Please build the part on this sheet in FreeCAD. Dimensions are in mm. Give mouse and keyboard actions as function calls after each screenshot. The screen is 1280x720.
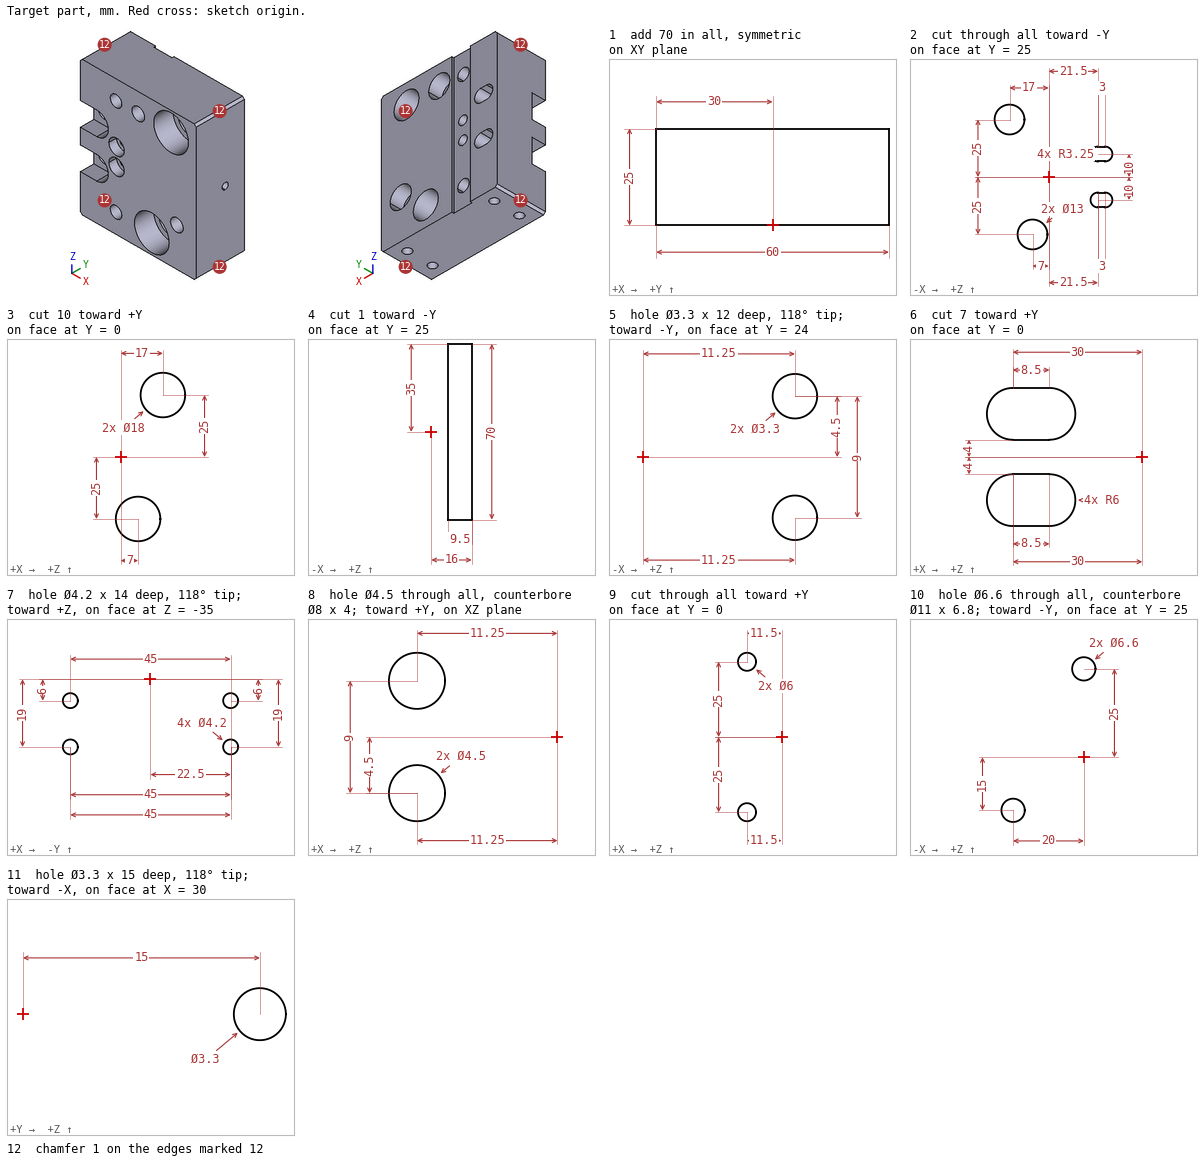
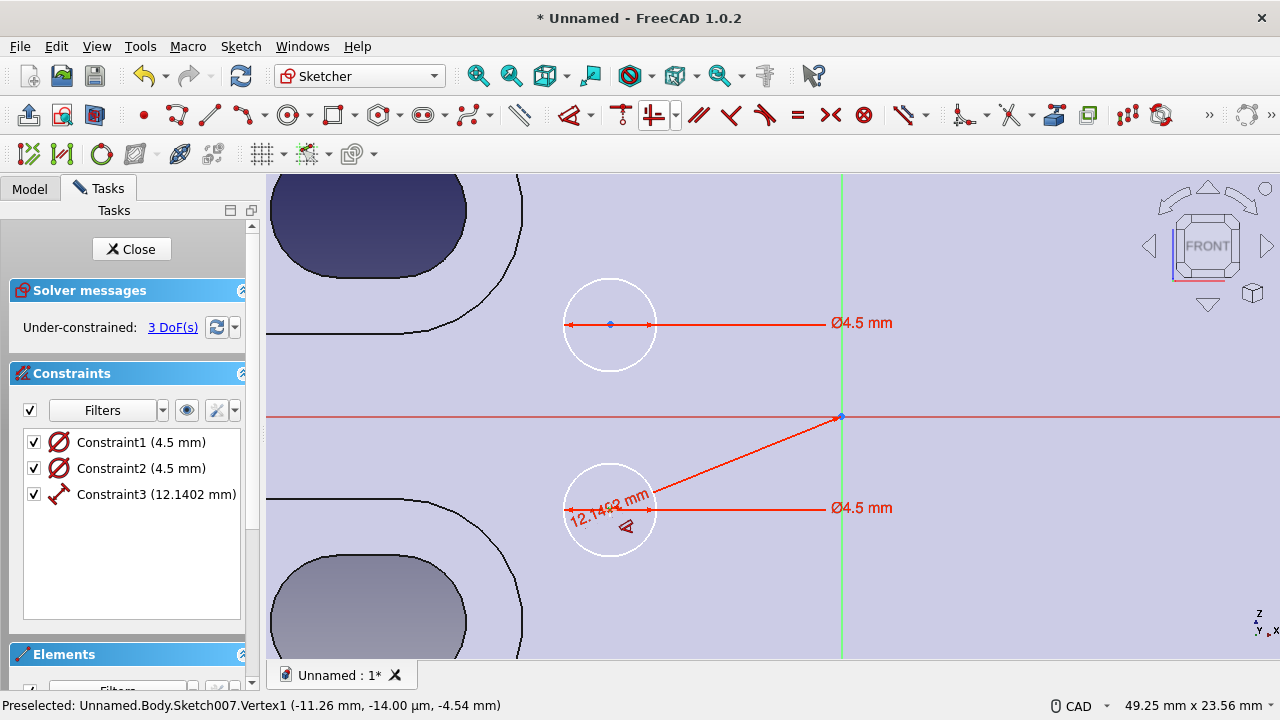
click(610, 325)
click(576, 375)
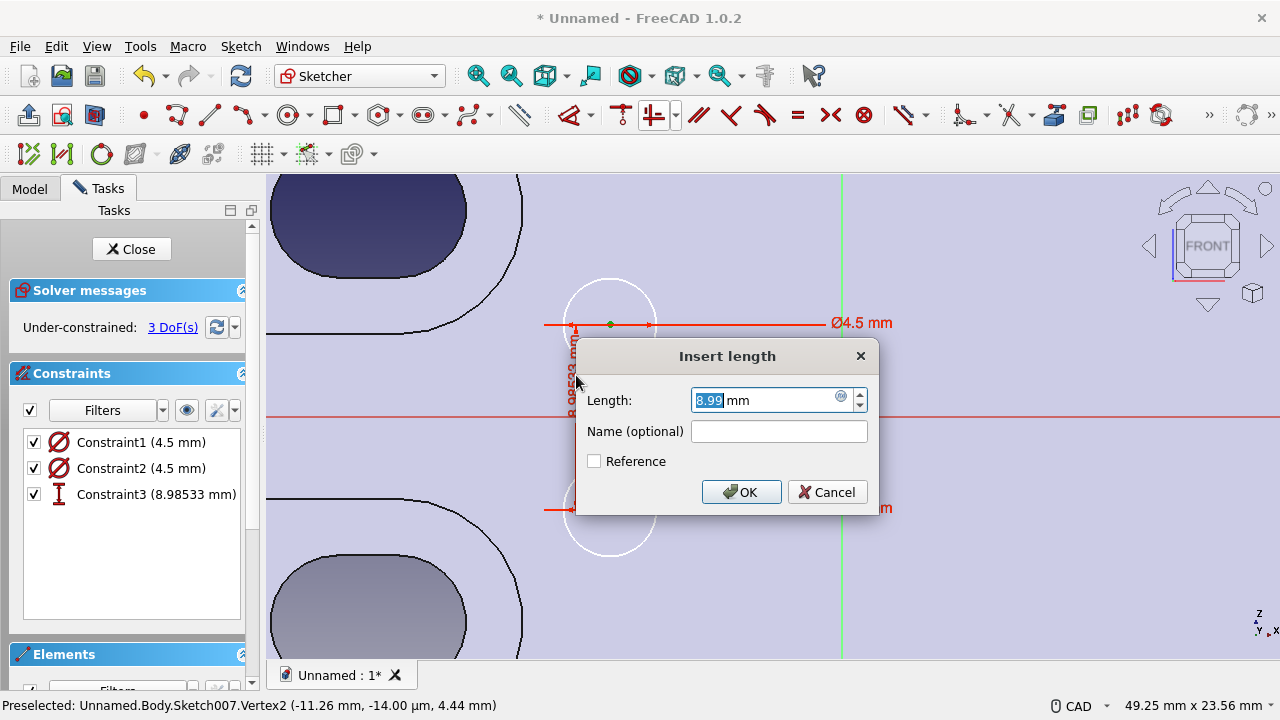
text(9)
key(Return)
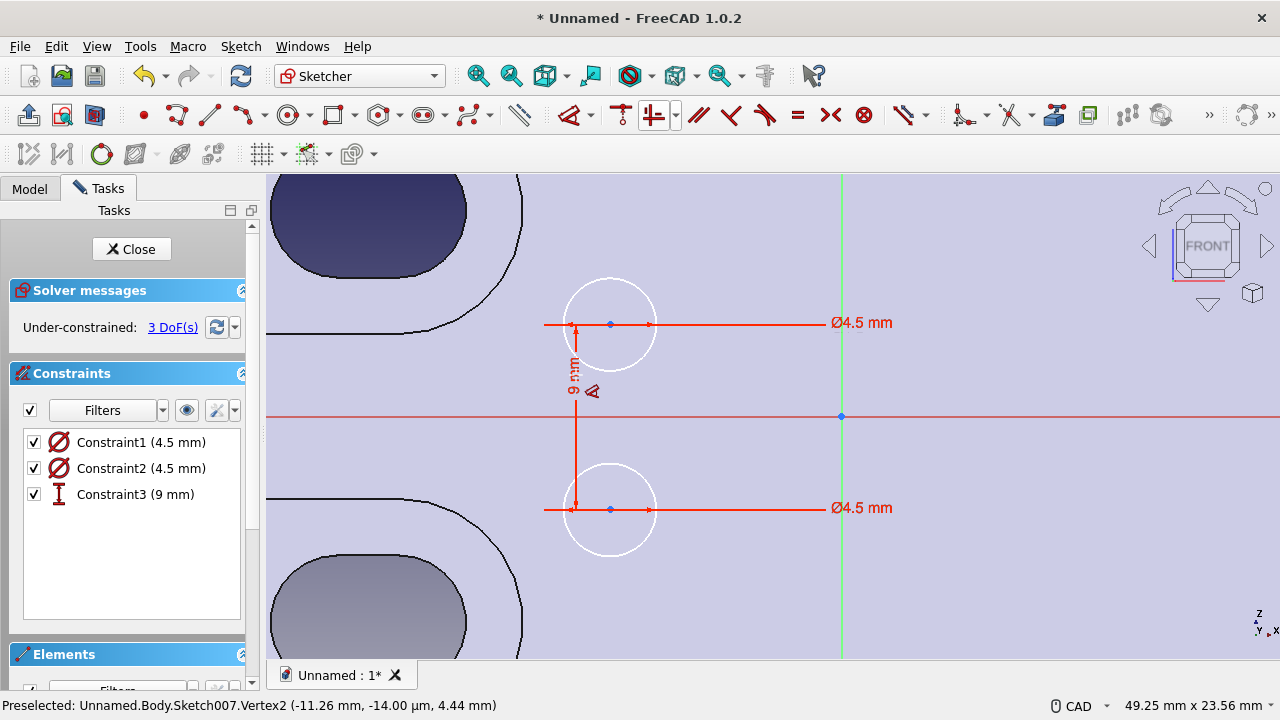
click(610, 510)
click(876, 463)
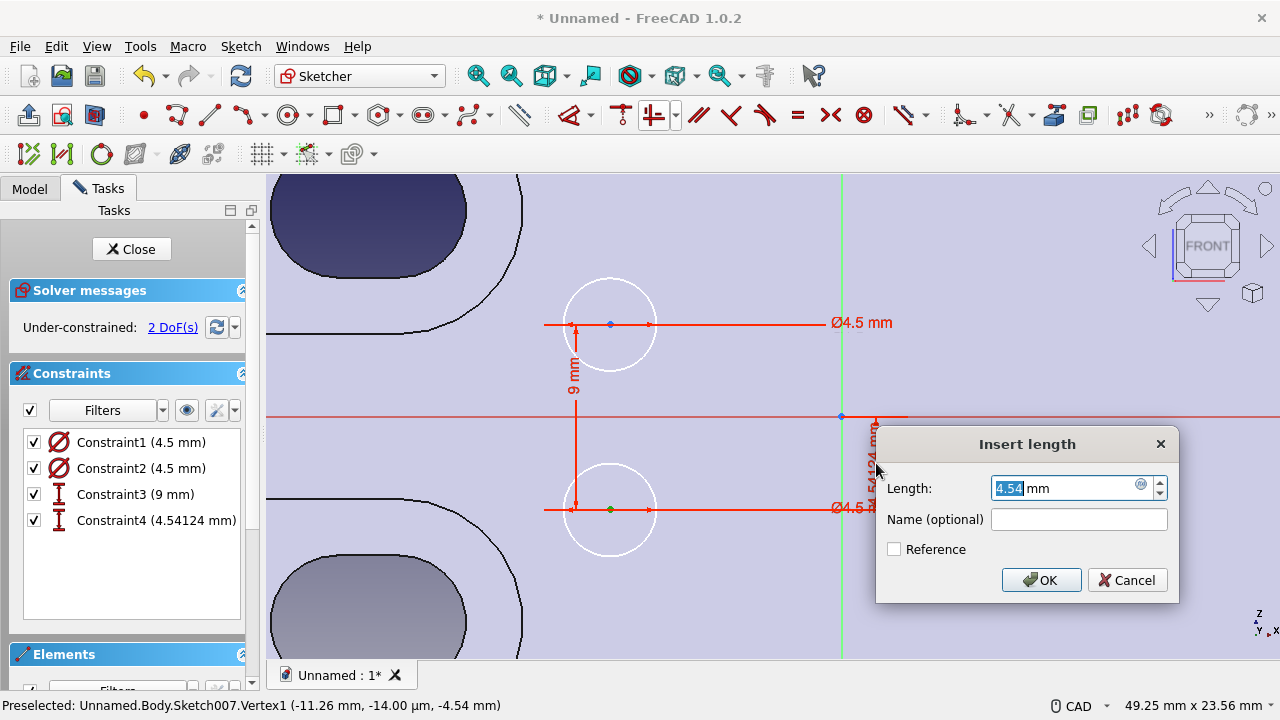
text(4.5)
key(Return)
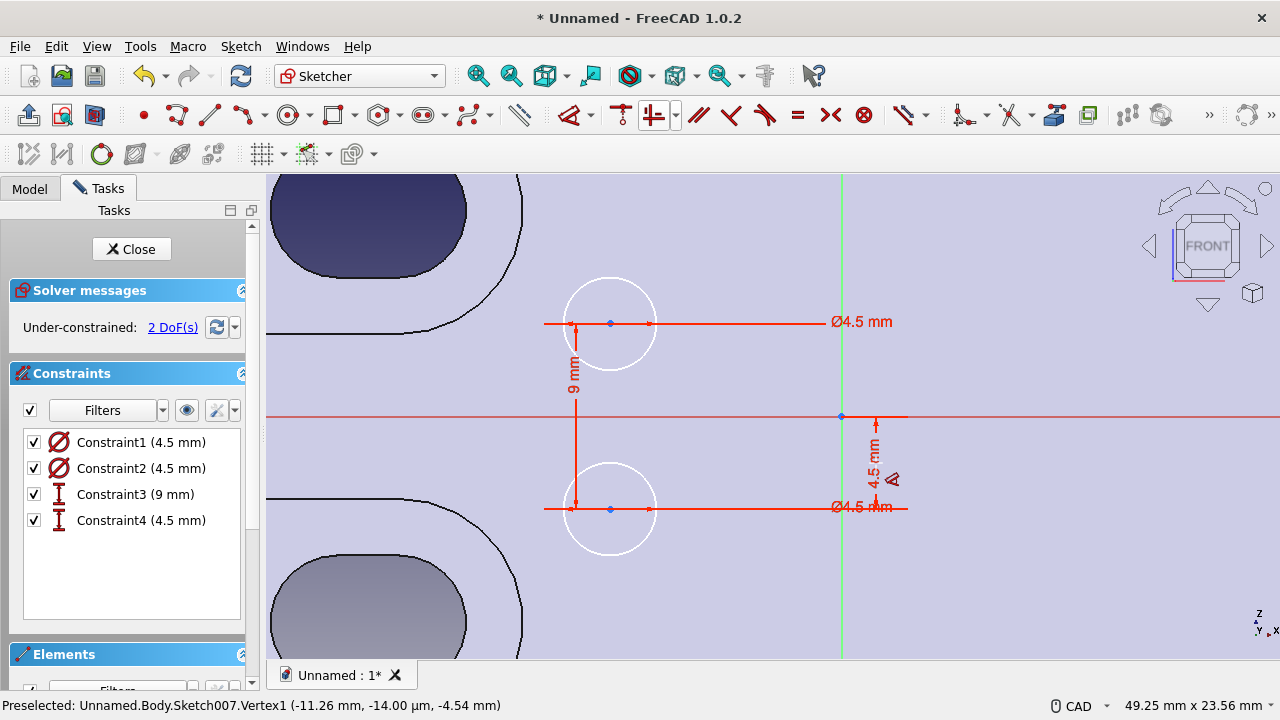
click(610, 509)
click(726, 543)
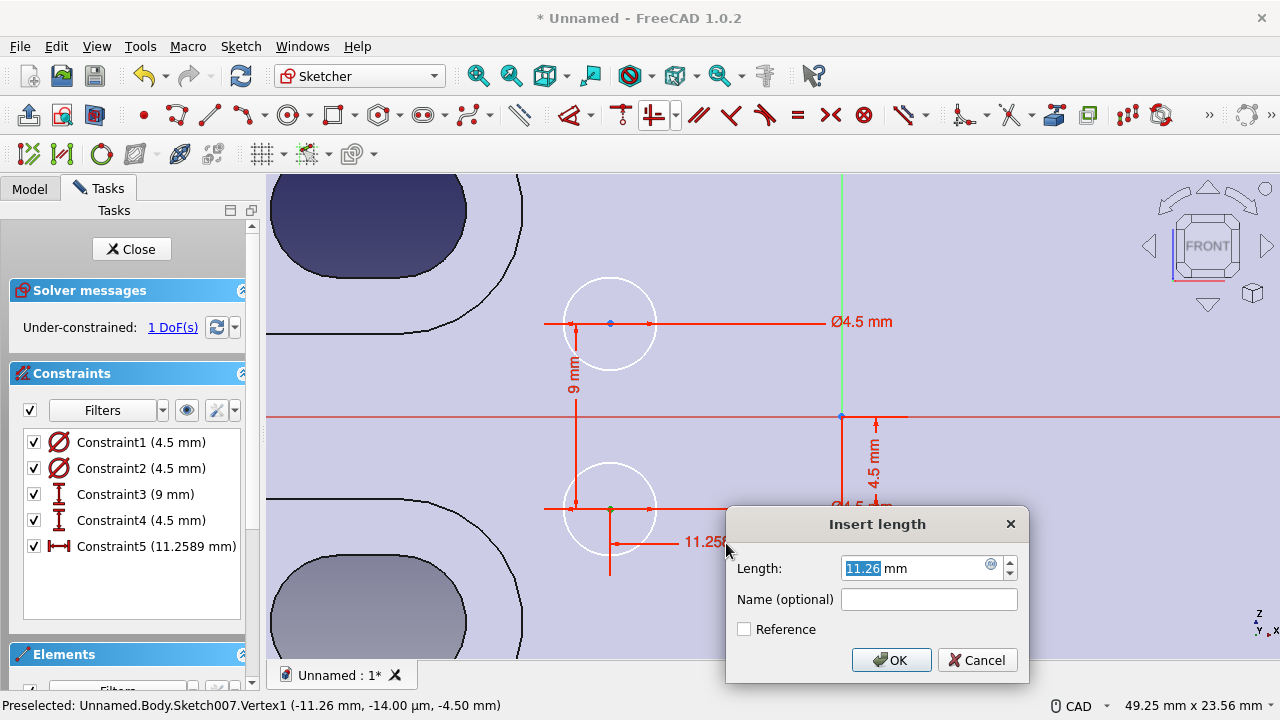
text(11.25)
key(Return)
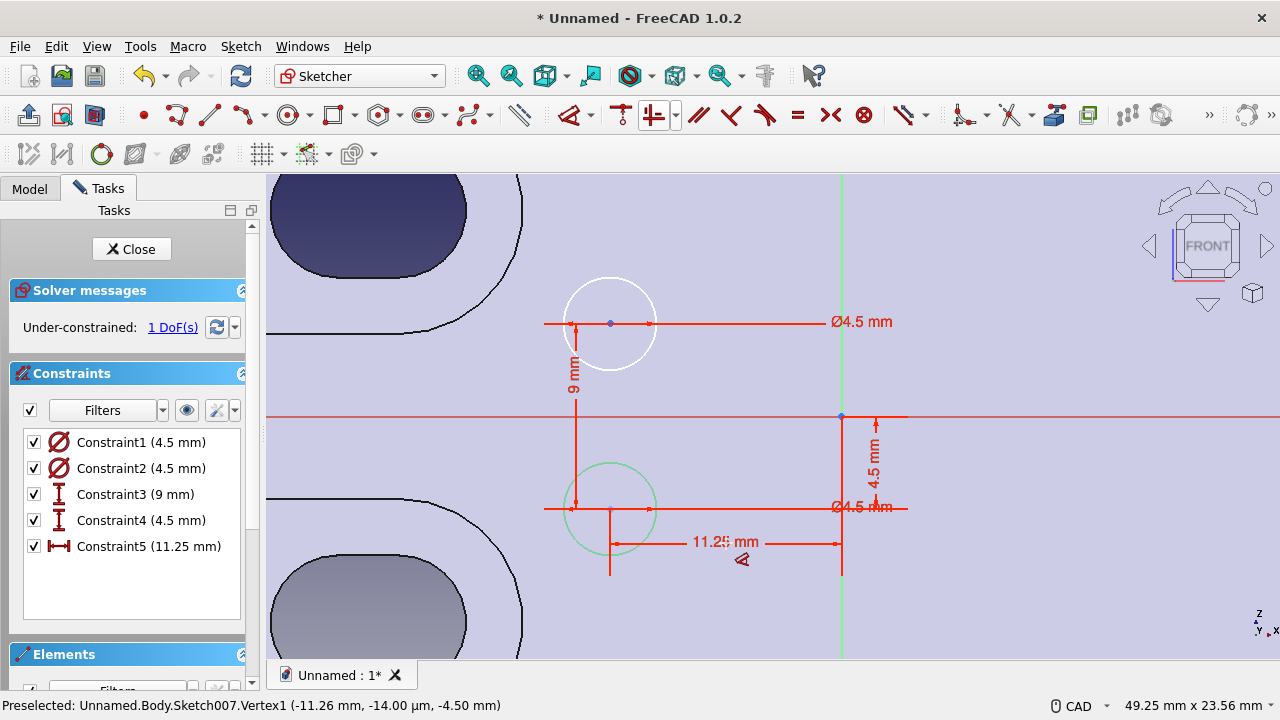
click(610, 324)
click(726, 290)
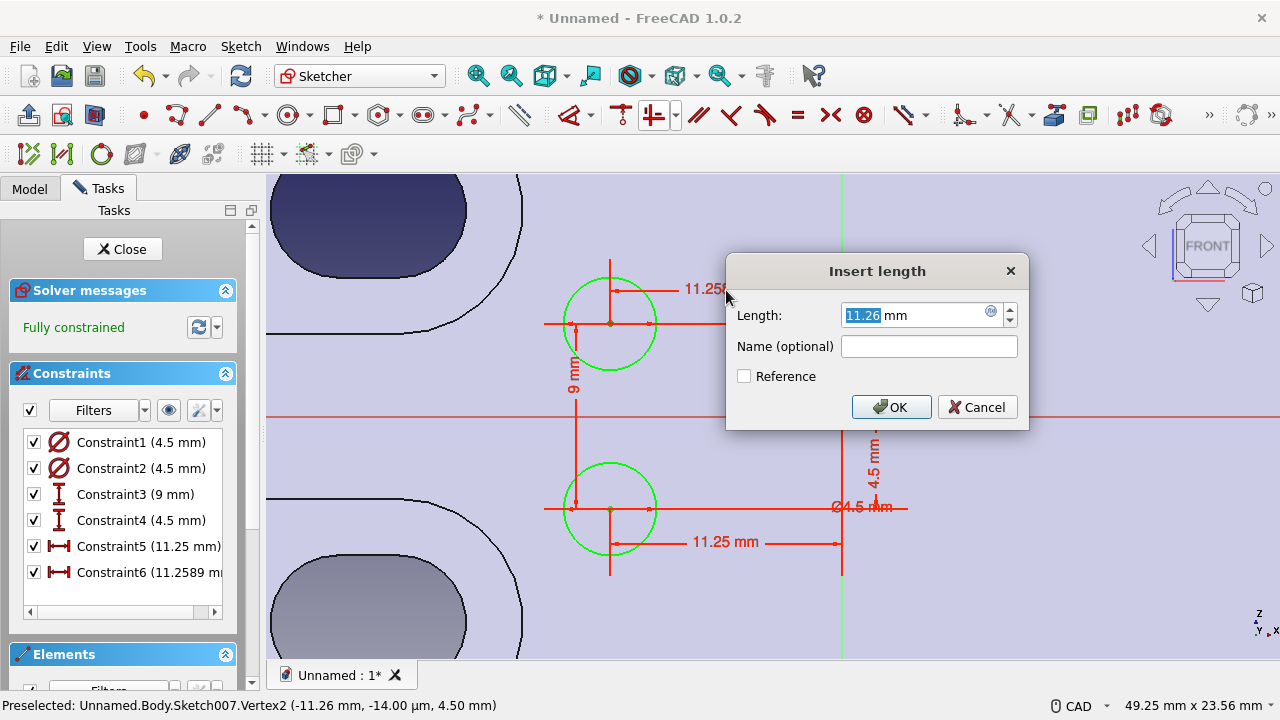
text(11.25)
key(Return)
key(Escape)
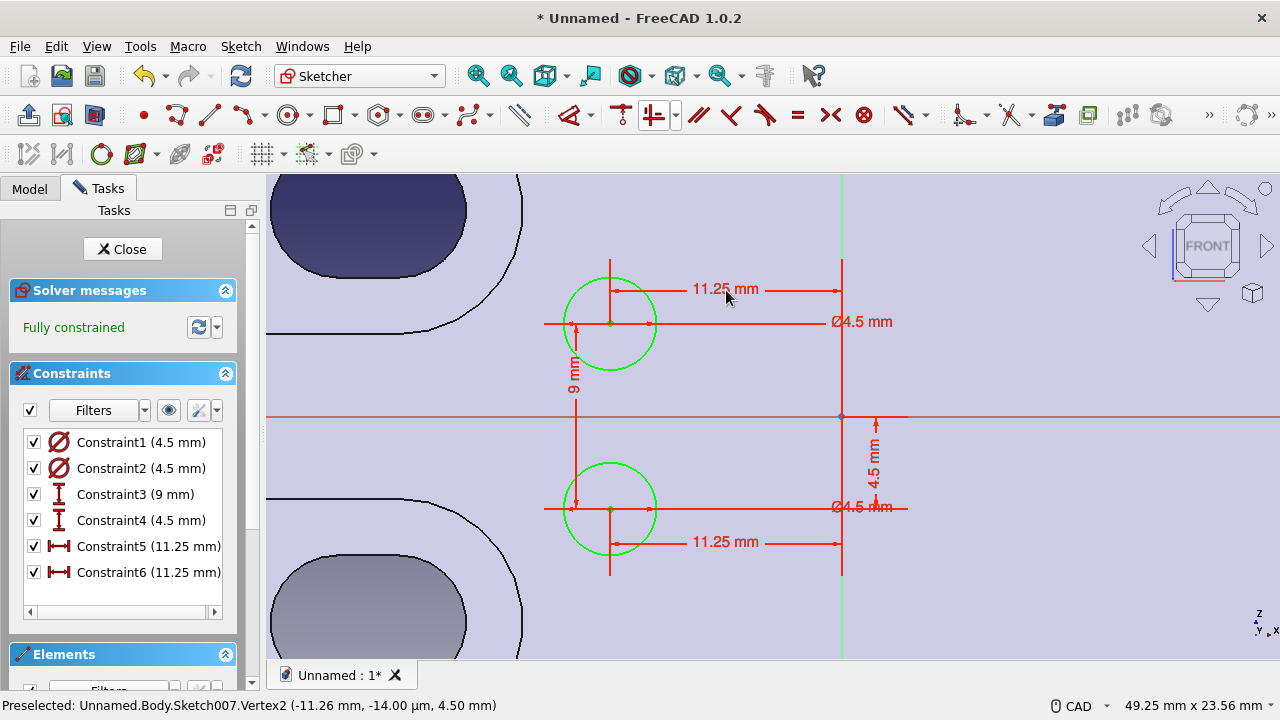
click(123, 249)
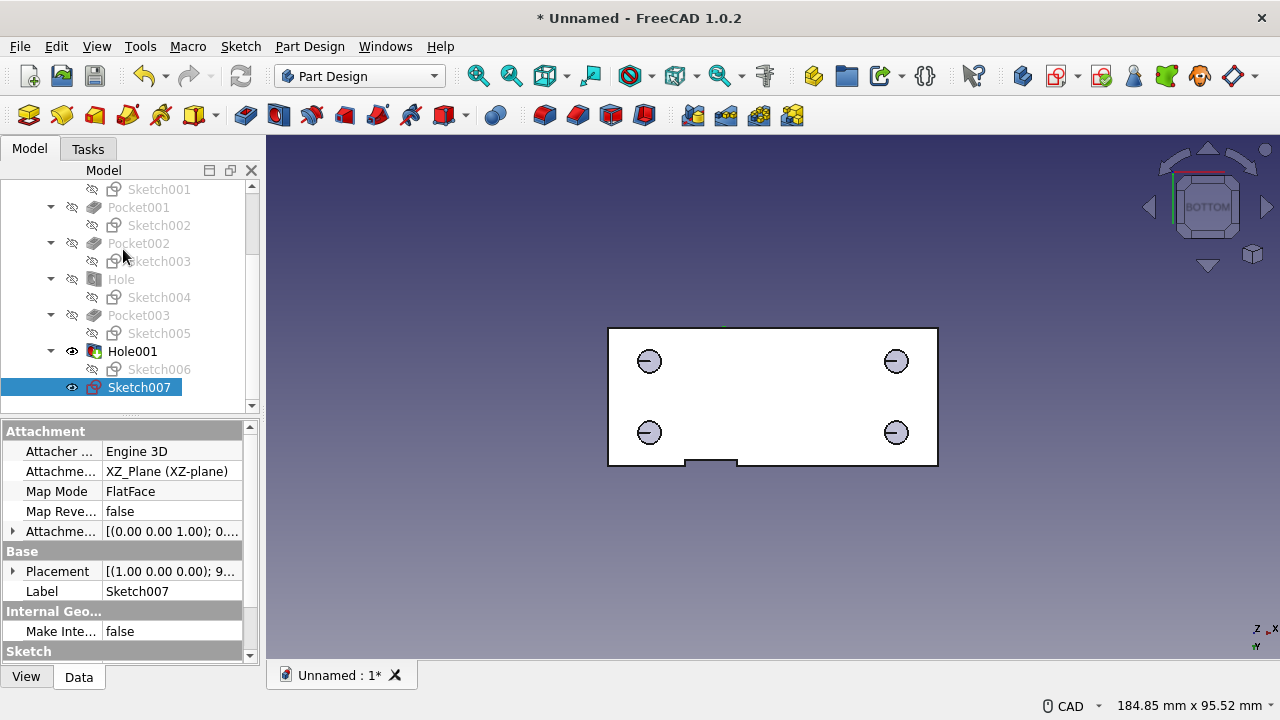
click(279, 116)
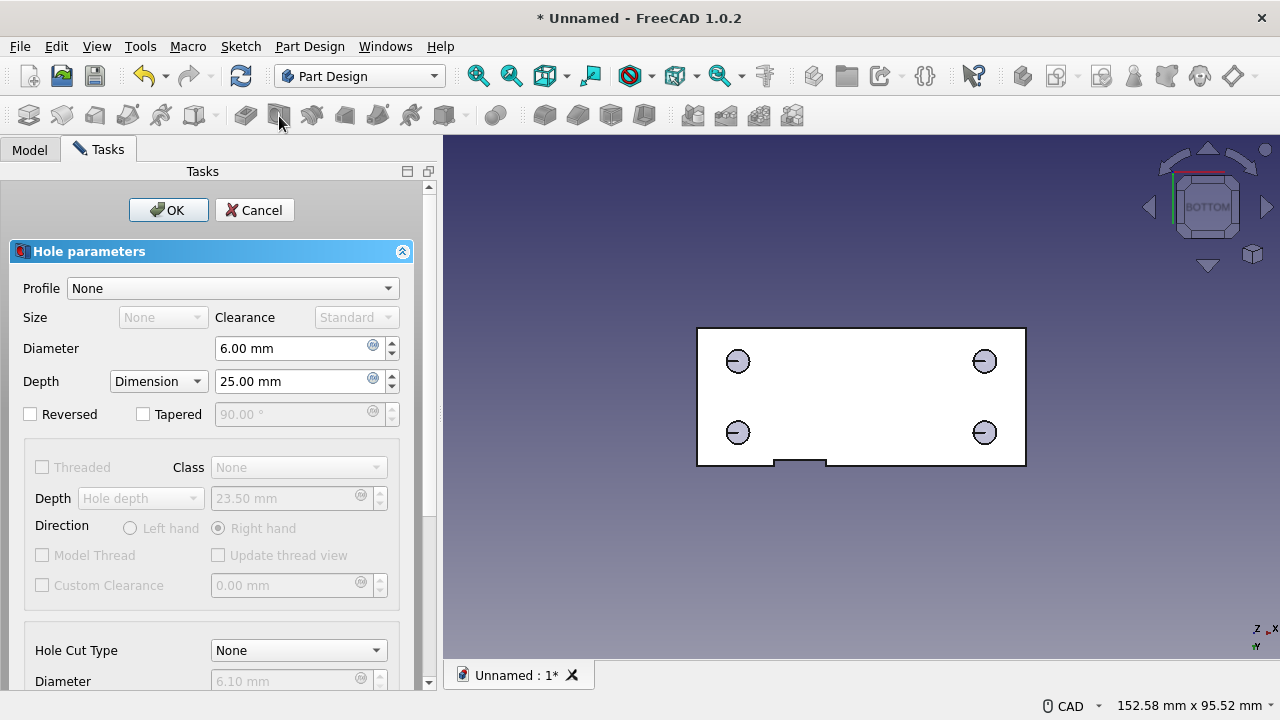
triple_click(300, 348)